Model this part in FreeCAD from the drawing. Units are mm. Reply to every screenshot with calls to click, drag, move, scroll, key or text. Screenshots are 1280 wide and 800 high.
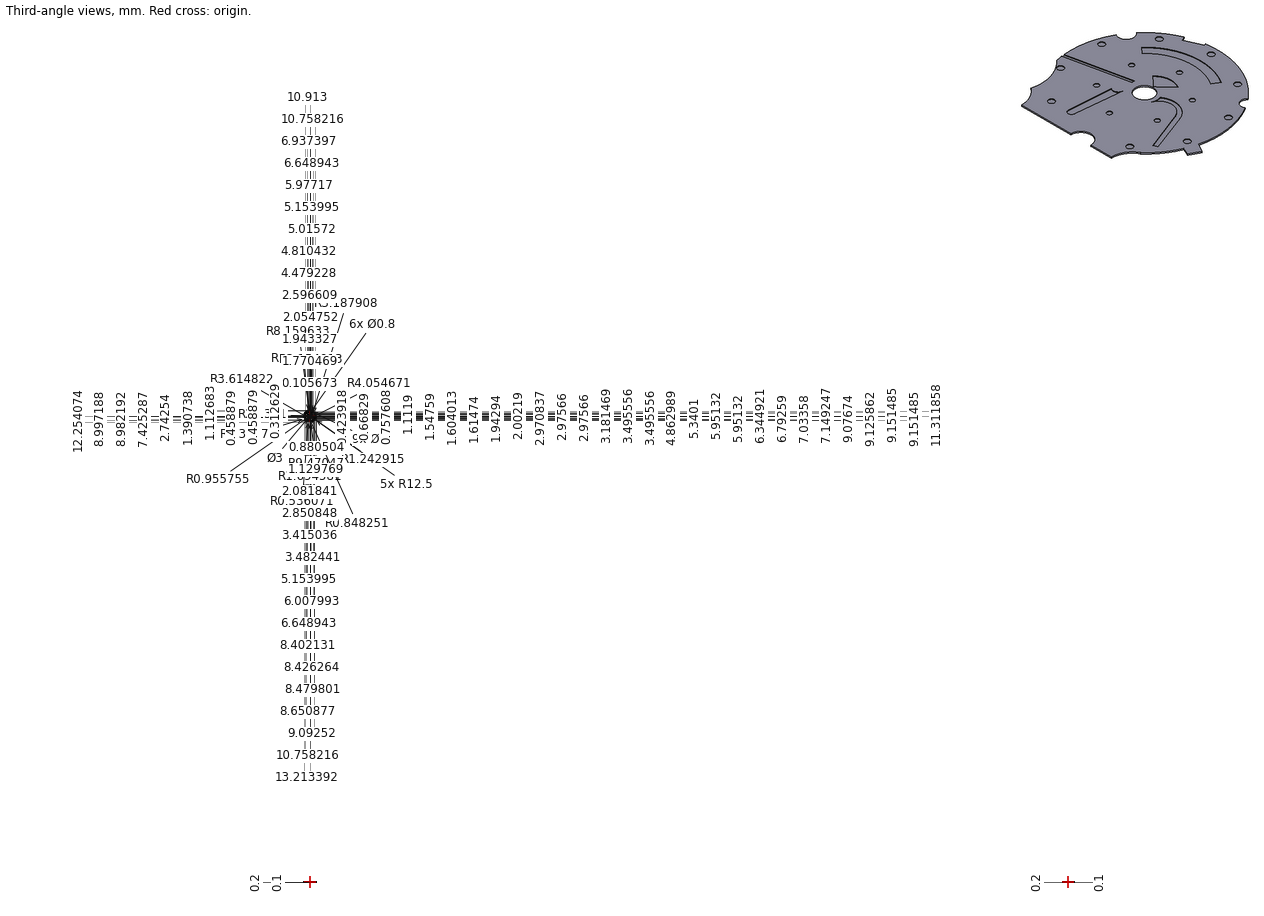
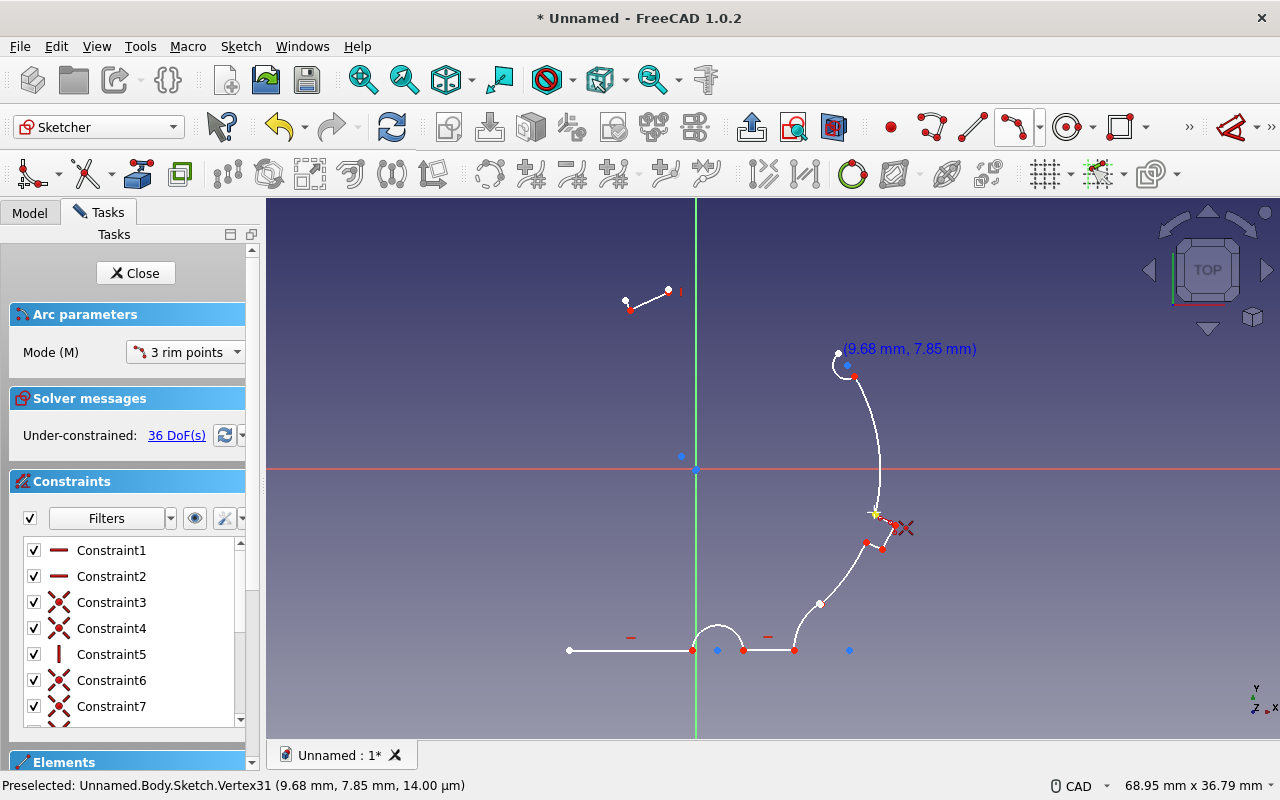
scroll(668, 288, up, 10)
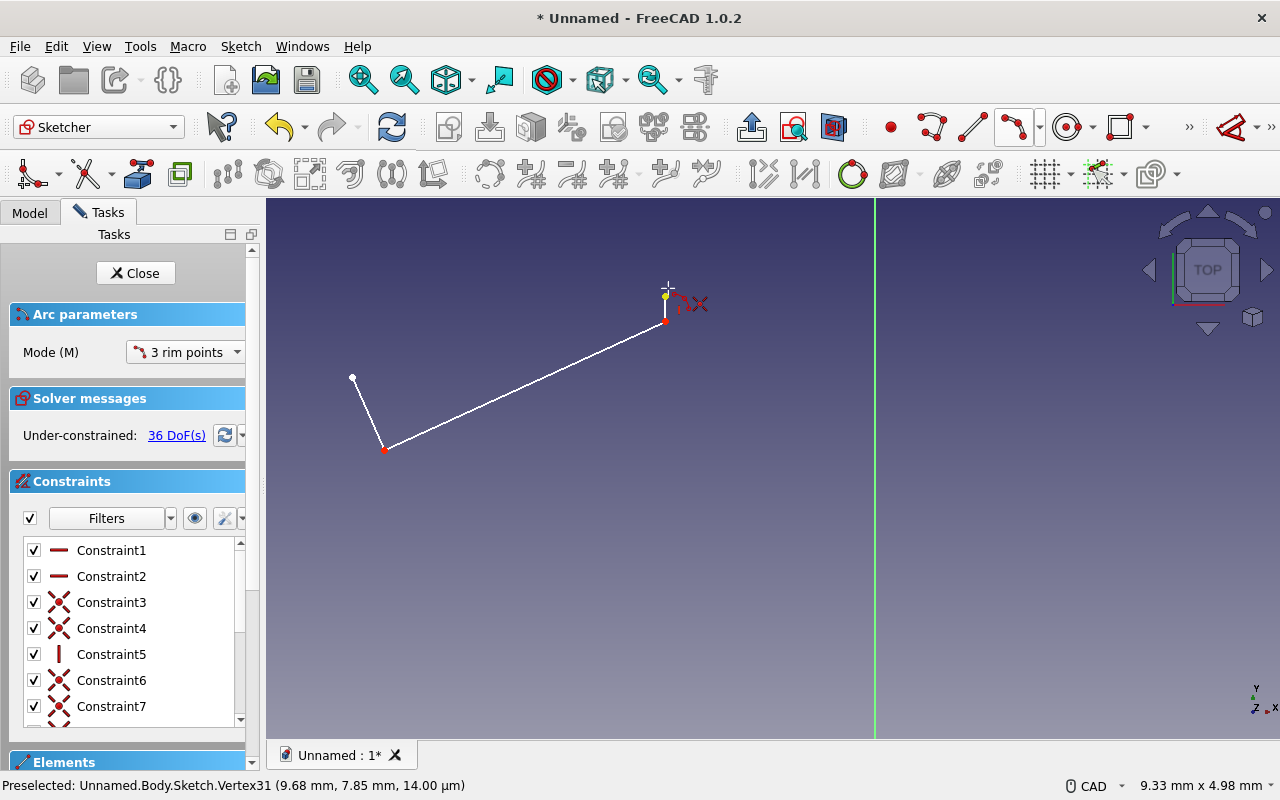
click(665, 297)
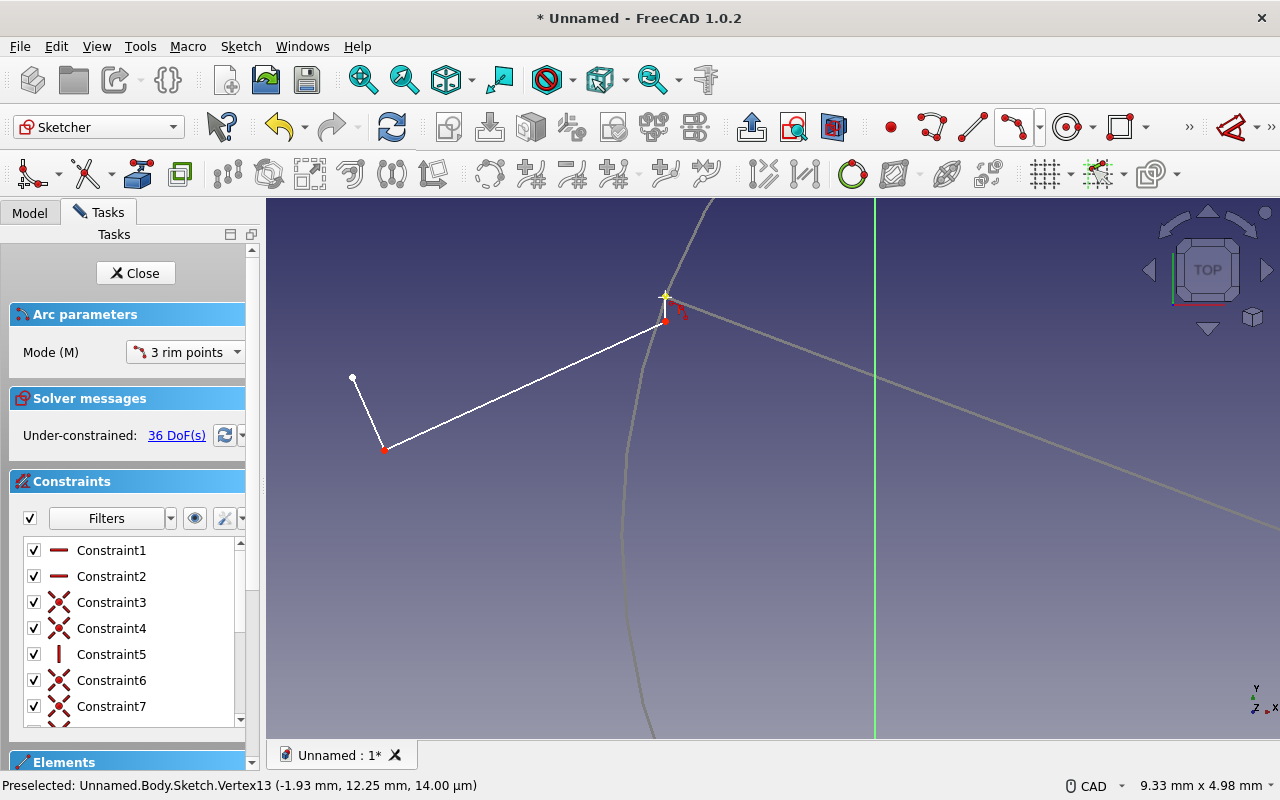
scroll(668, 288, down, 10)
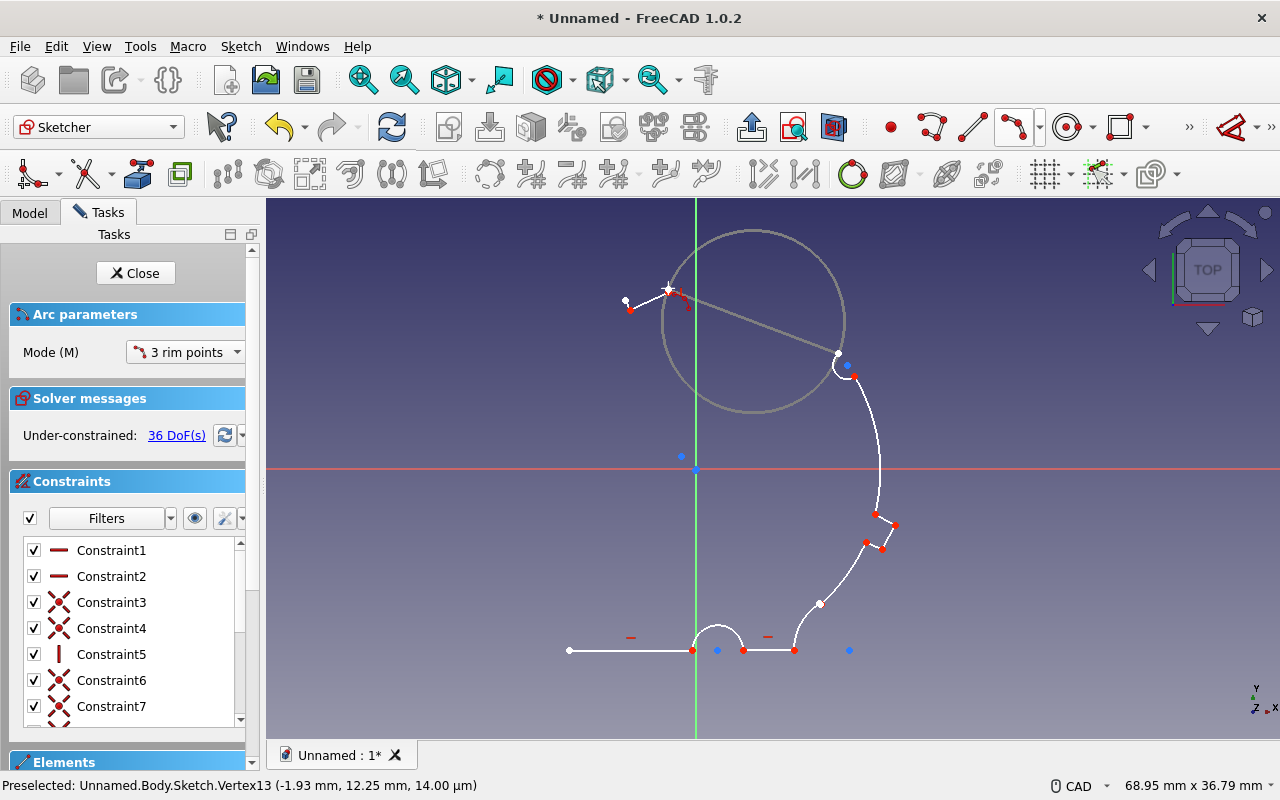
click(762, 298)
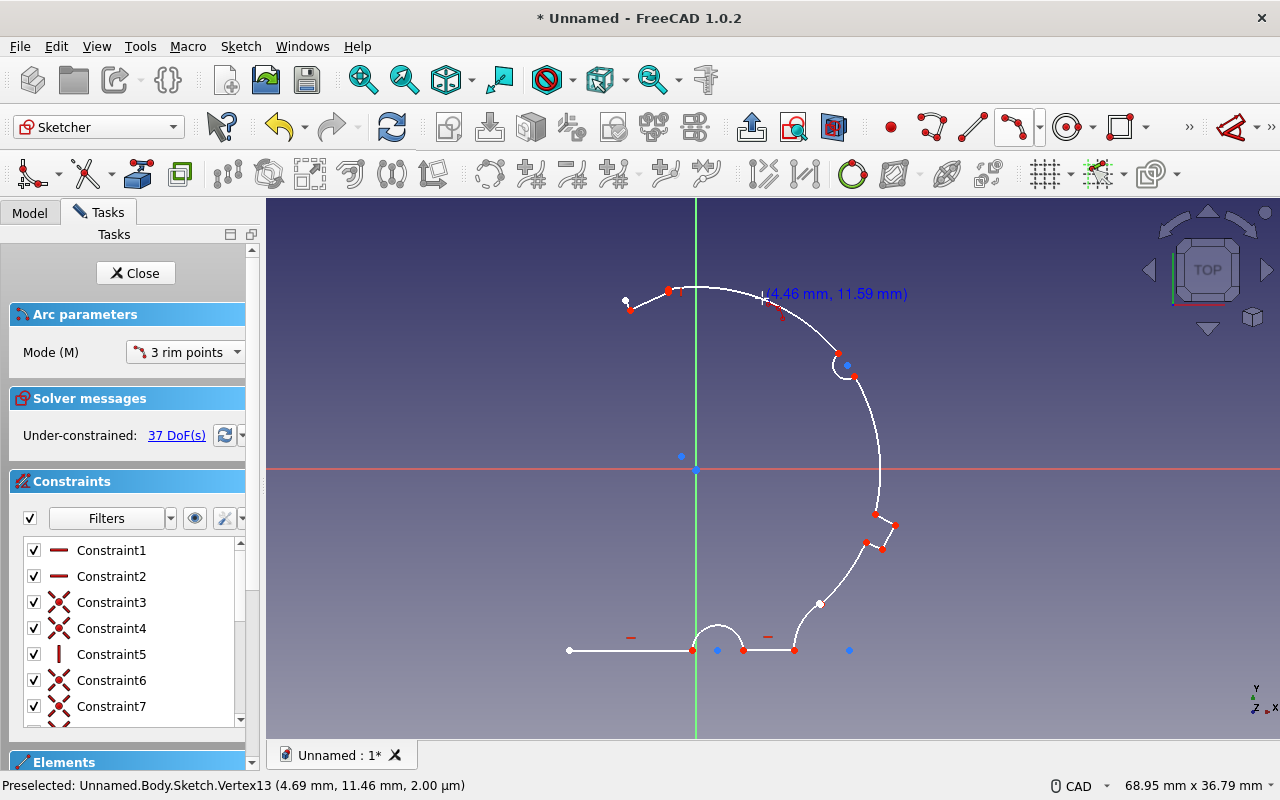
scroll(626, 300, up, 6)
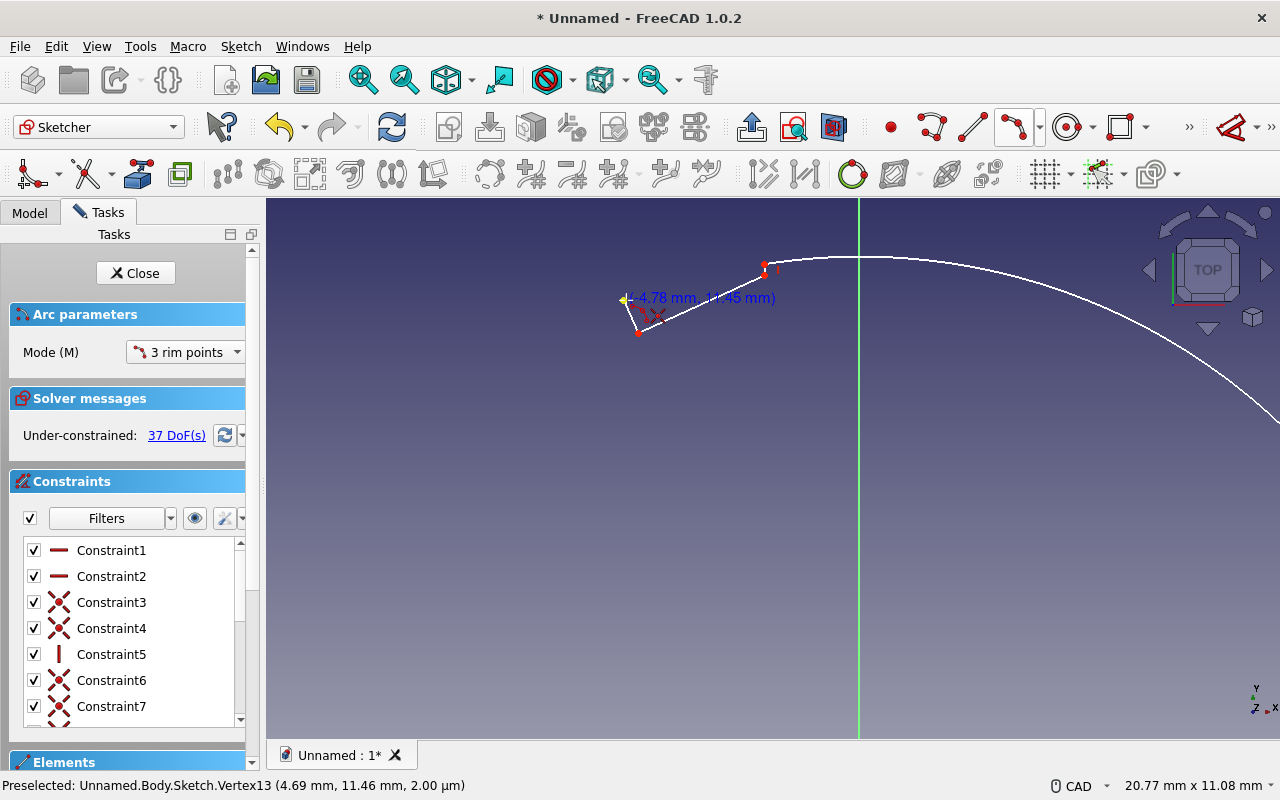
click(624, 300)
click(395, 465)
click(500, 369)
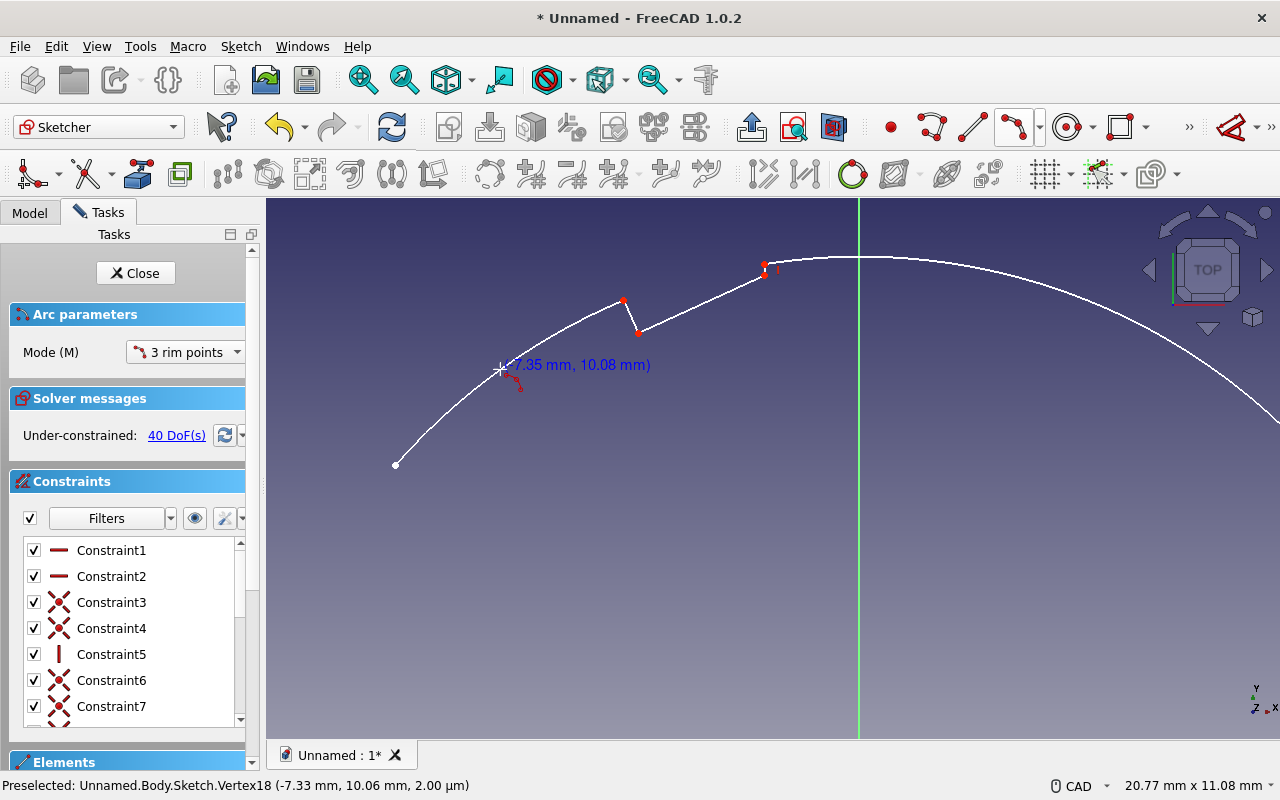
click(395, 466)
click(326, 565)
click(408, 548)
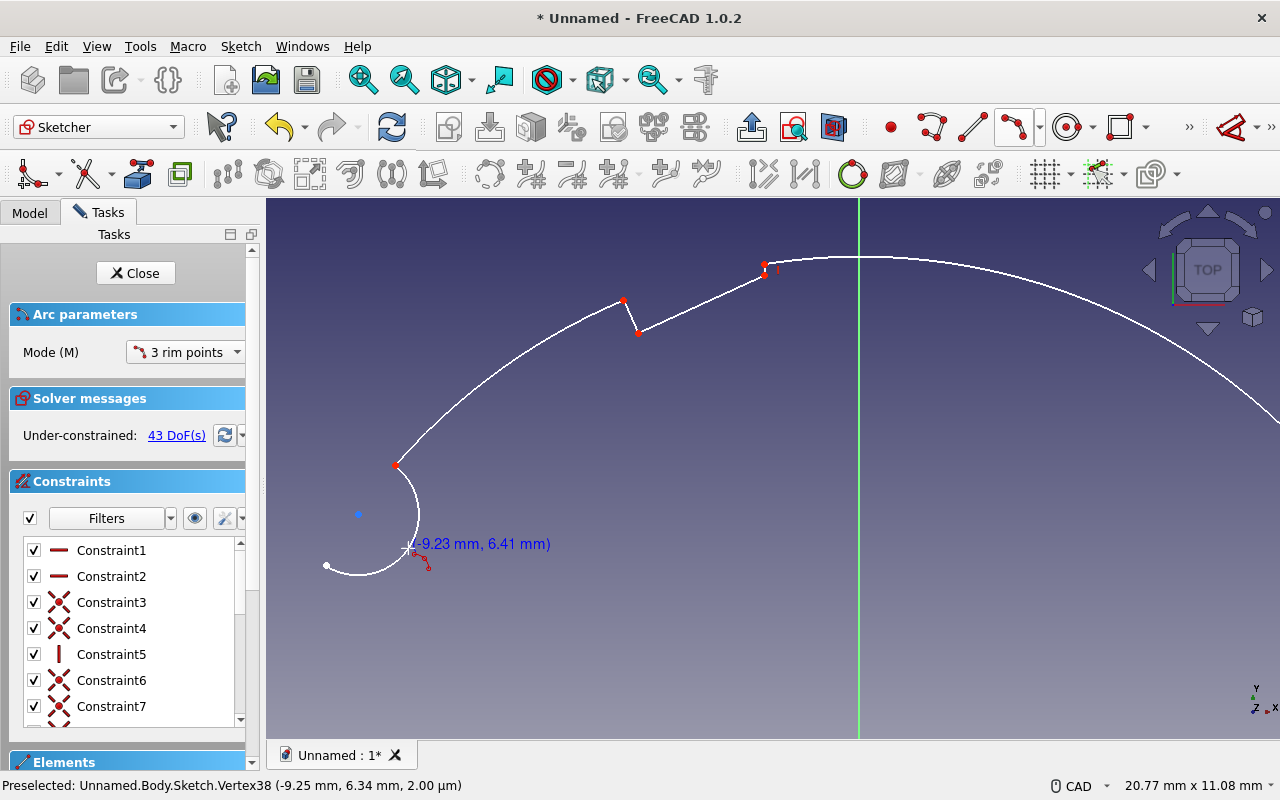
click(326, 566)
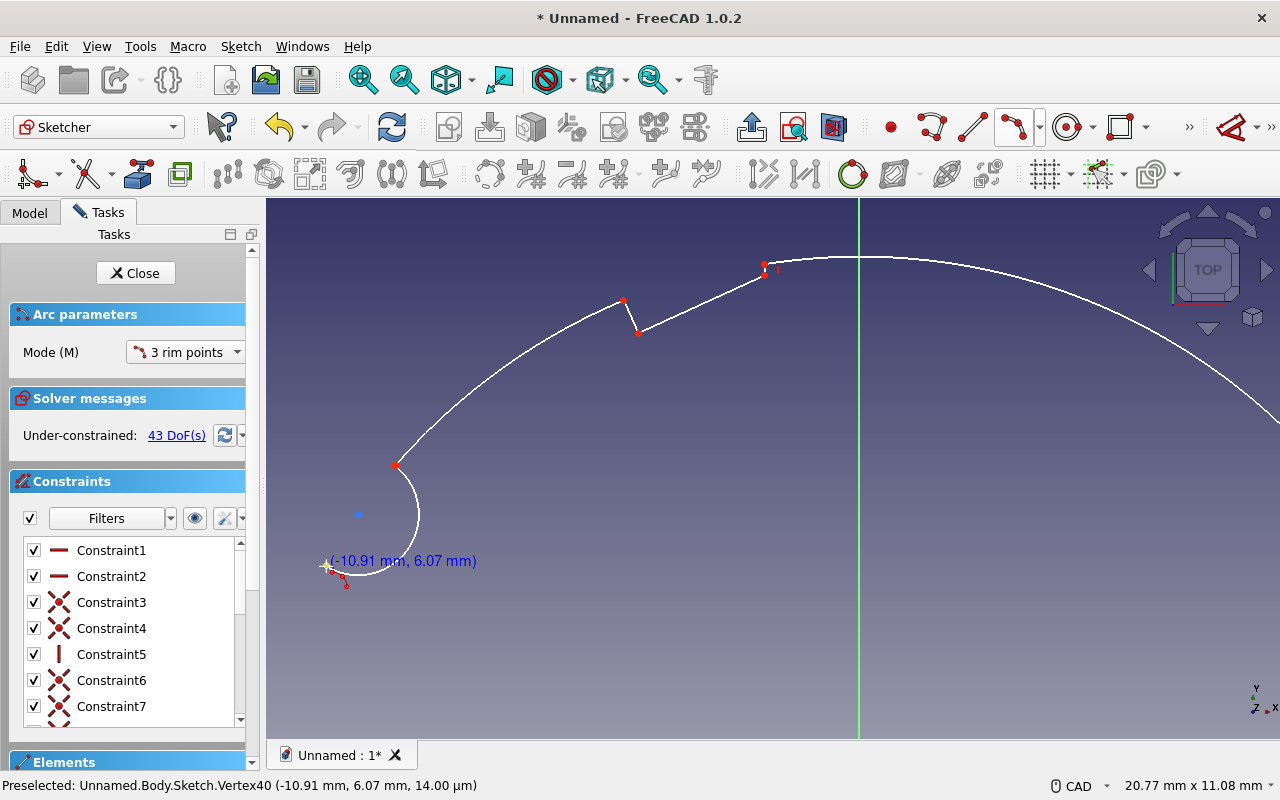
scroll(626, 300, down, 6)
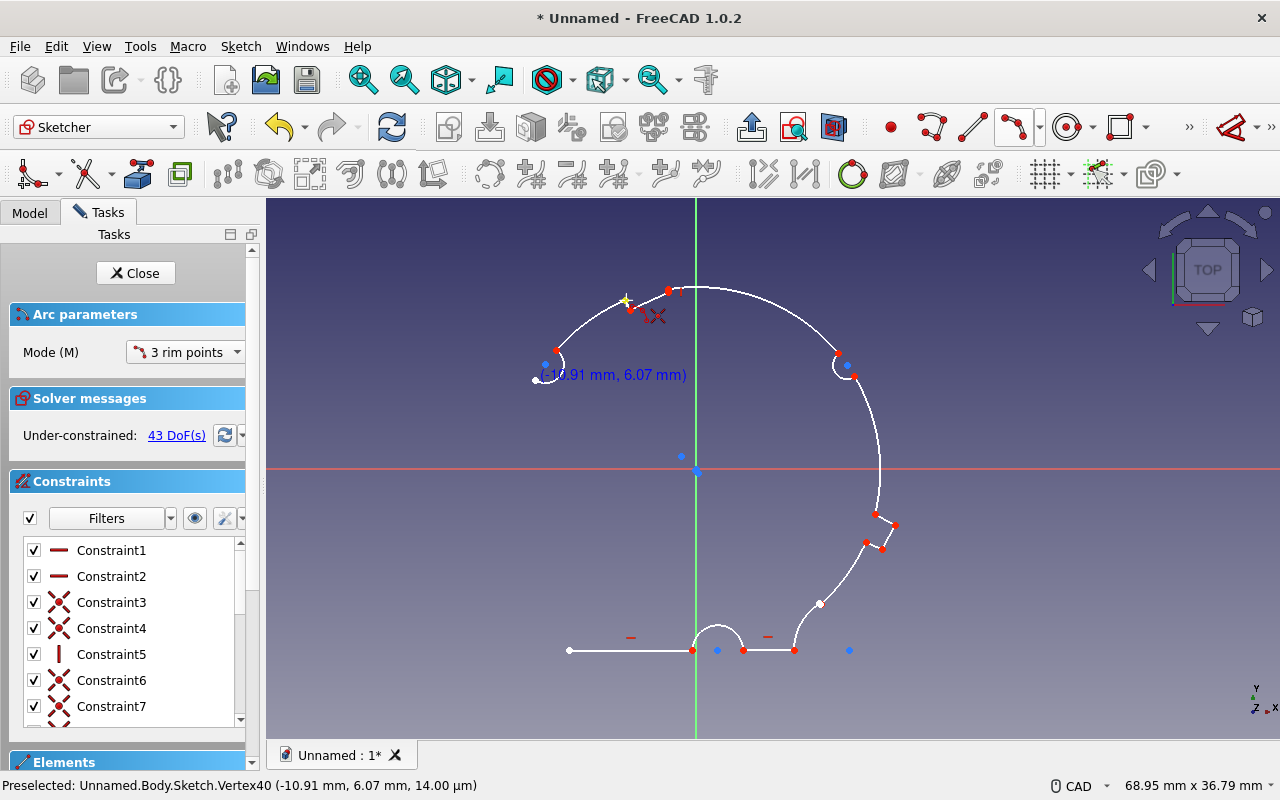
click(517, 510)